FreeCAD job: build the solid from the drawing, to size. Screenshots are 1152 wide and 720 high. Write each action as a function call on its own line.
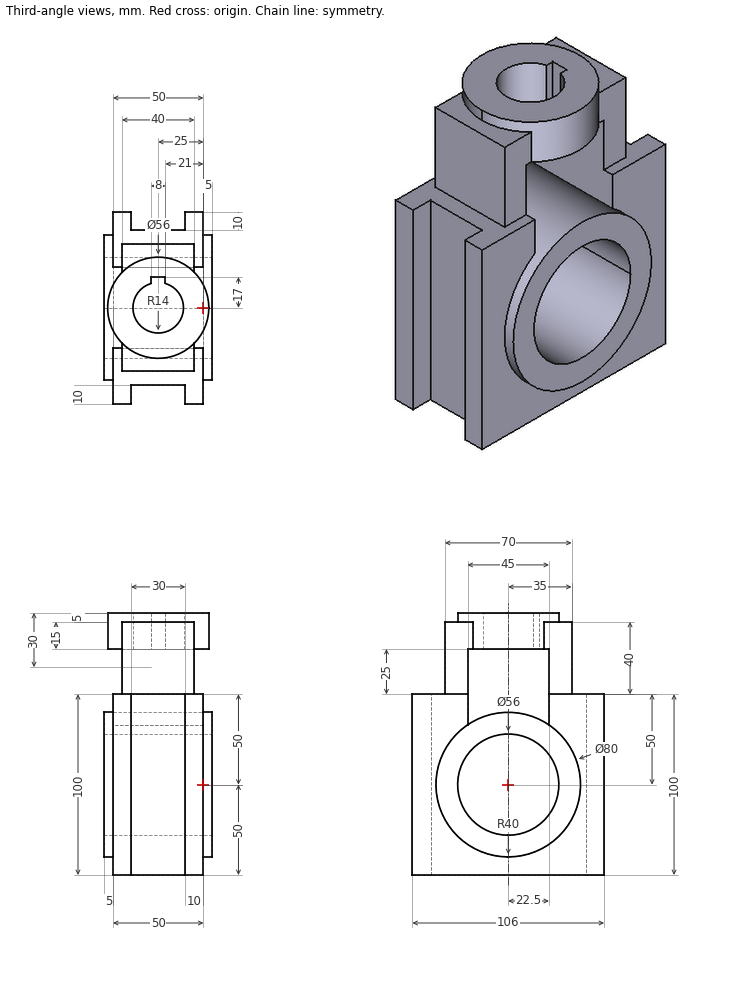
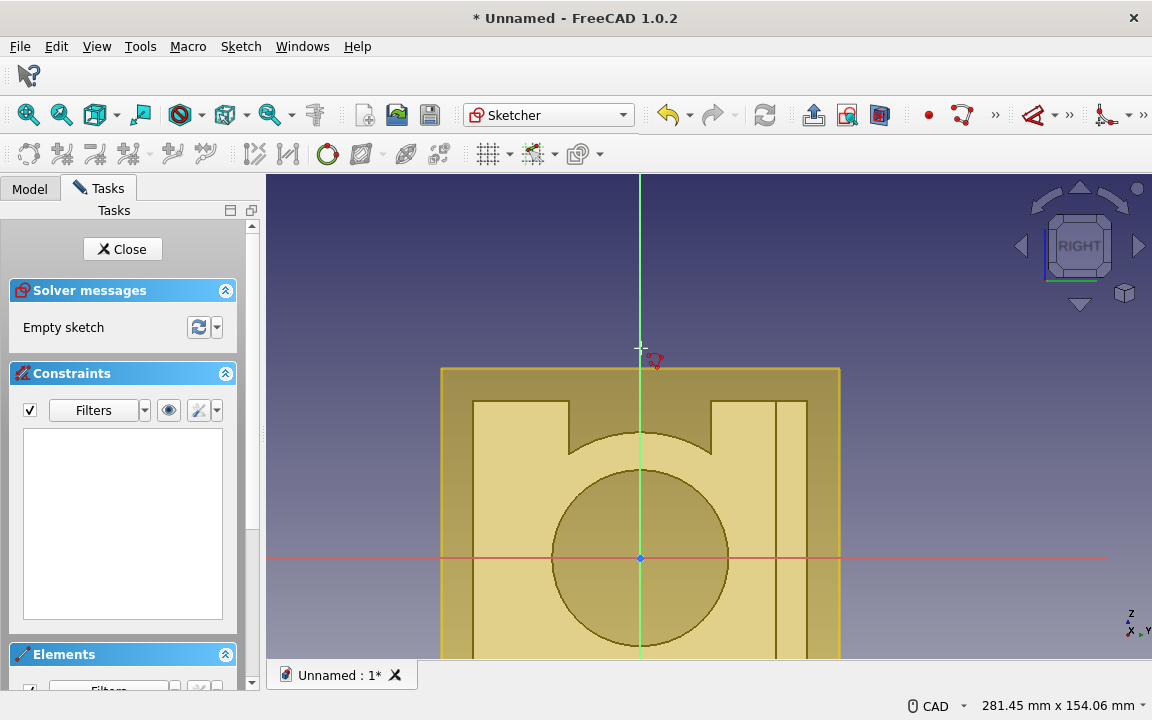
click(569, 401)
click(569, 322)
click(711, 322)
click(711, 401)
click(750, 401)
click(750, 275)
click(530, 275)
click(530, 401)
click(569, 402)
key(Escape)
key(Escape)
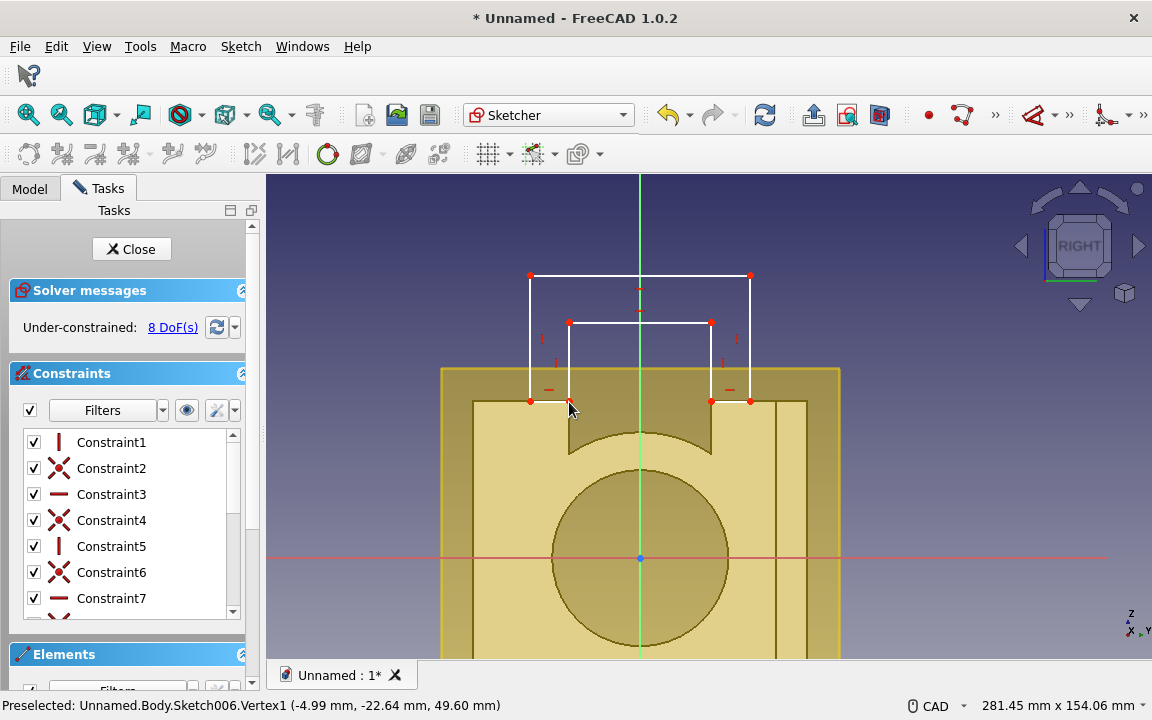
click(569, 402)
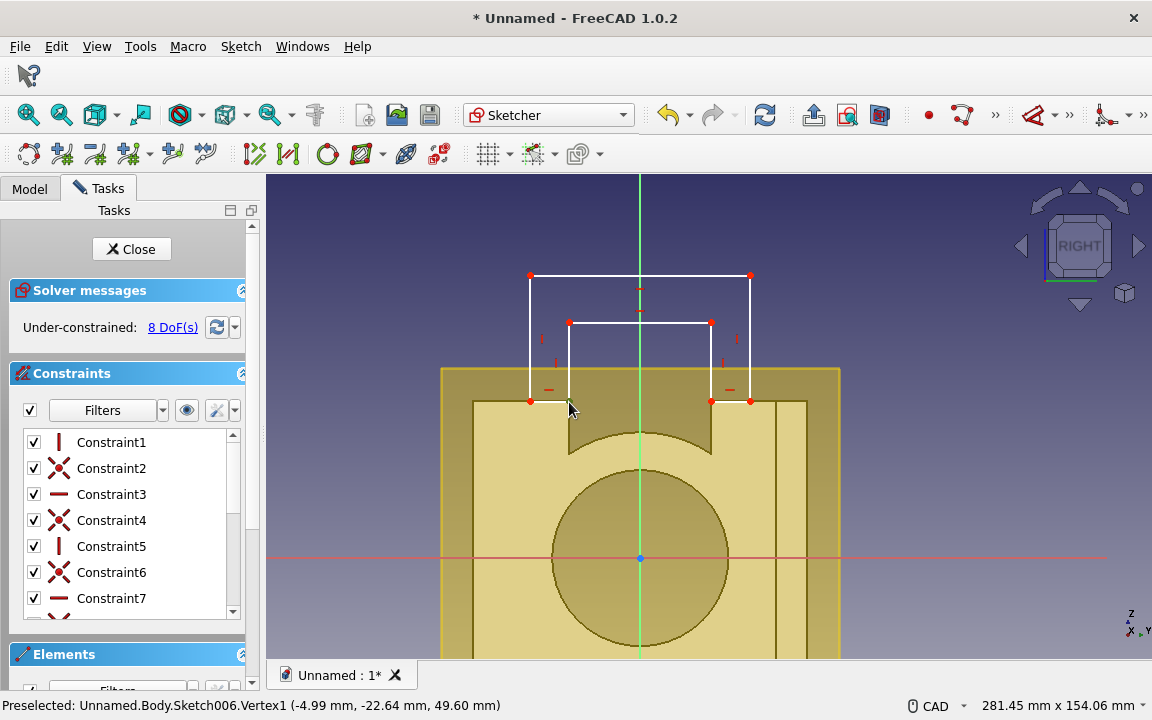
click(711, 402)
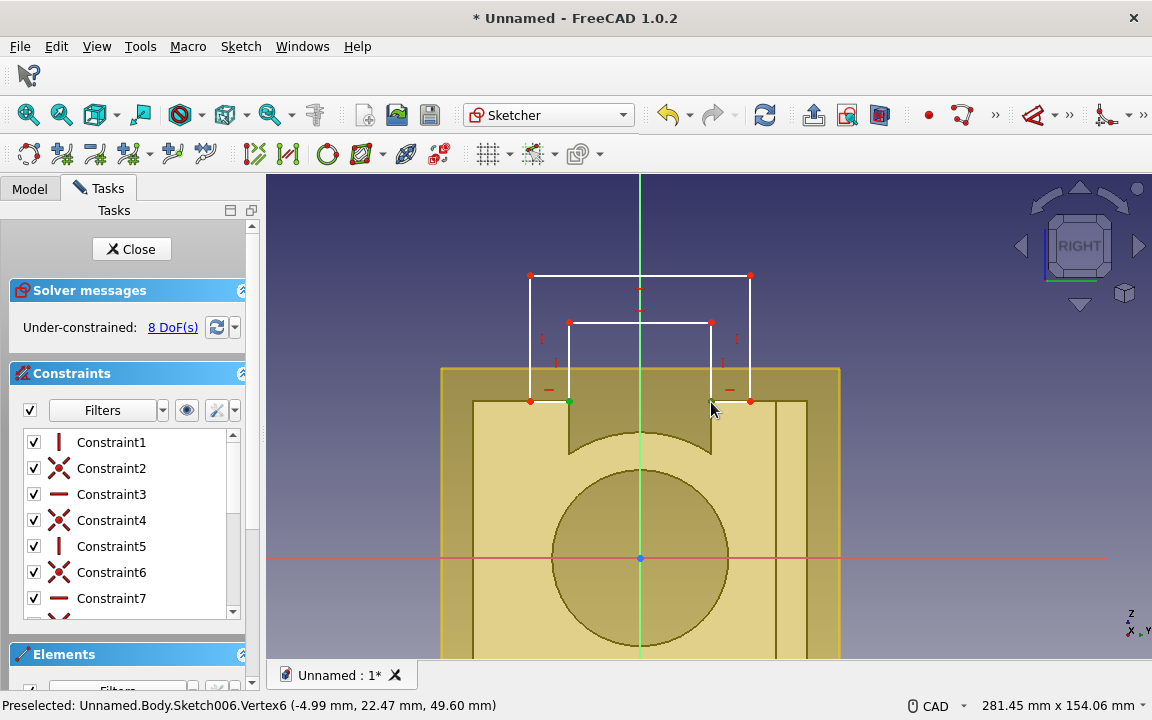
click(640, 600)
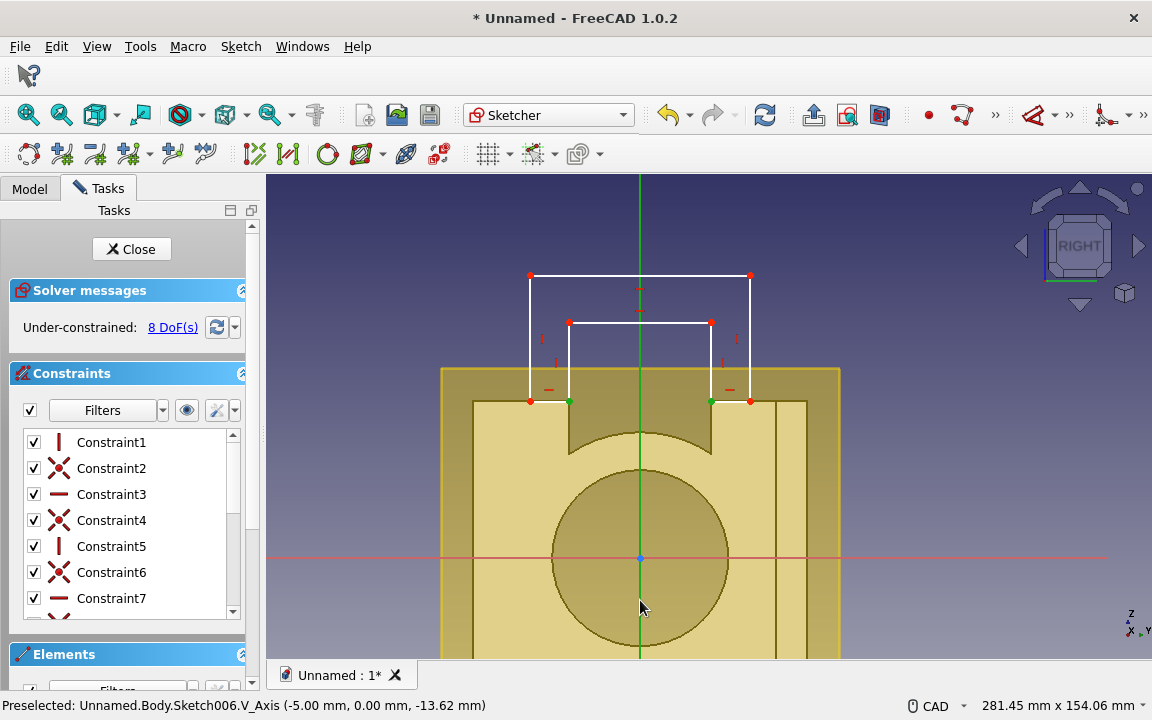
key(s)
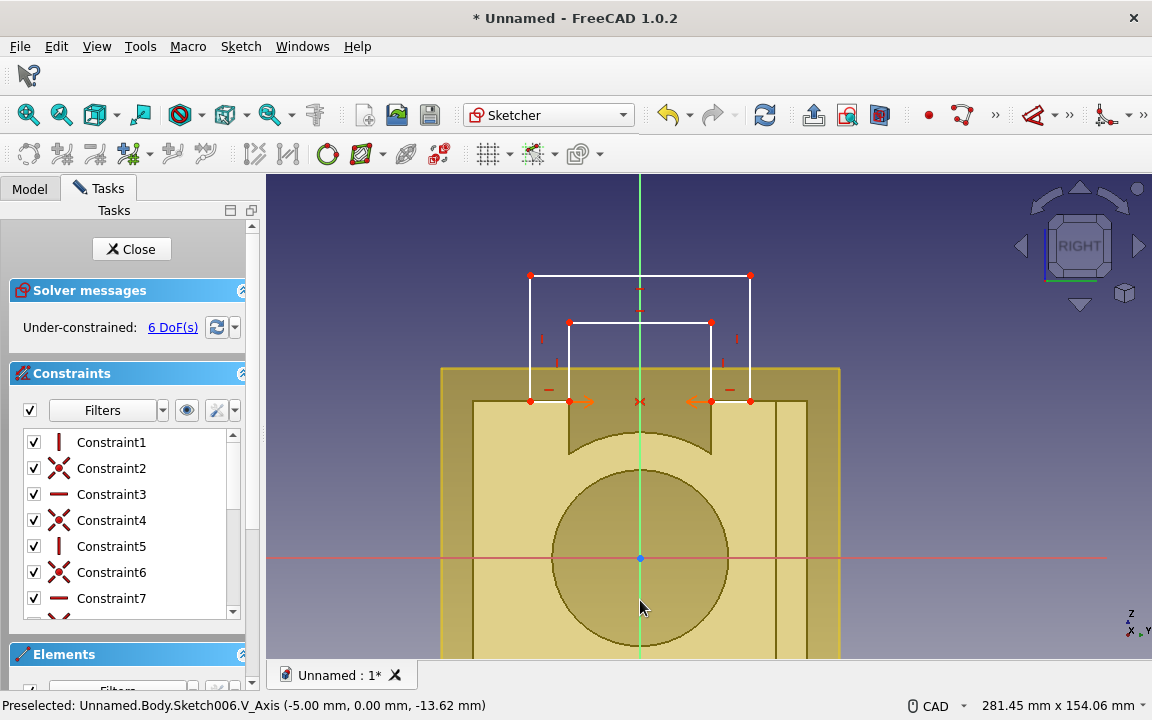
key(d)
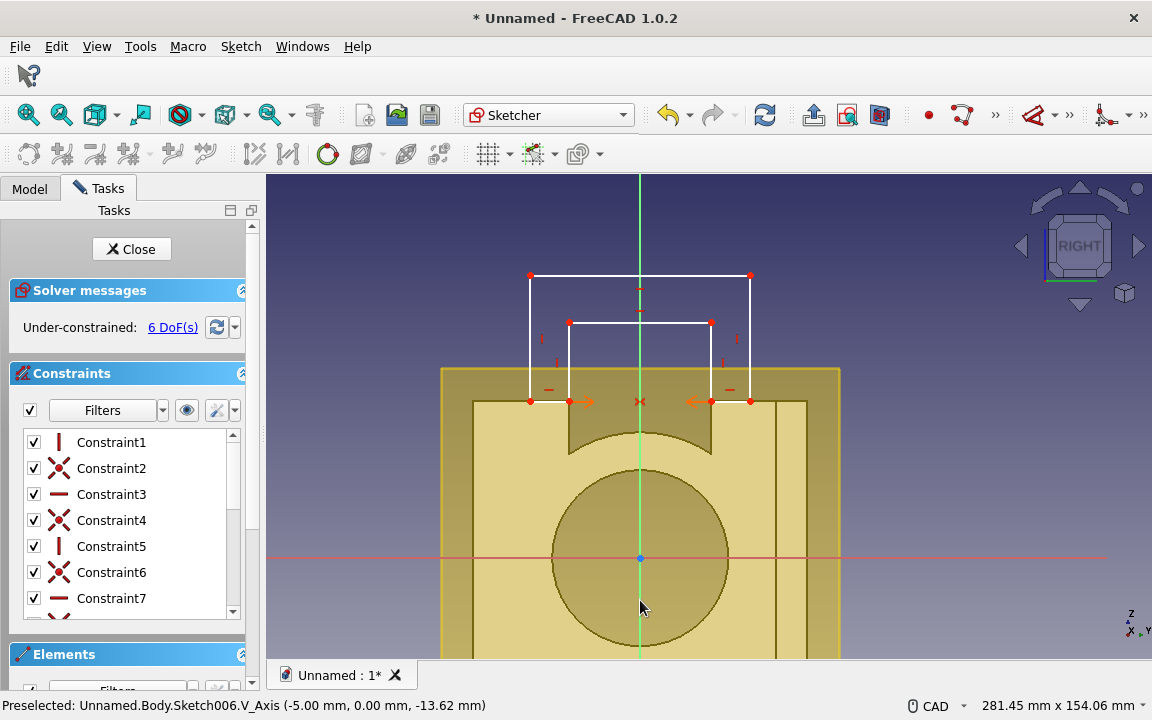
click(569, 378)
click(603, 362)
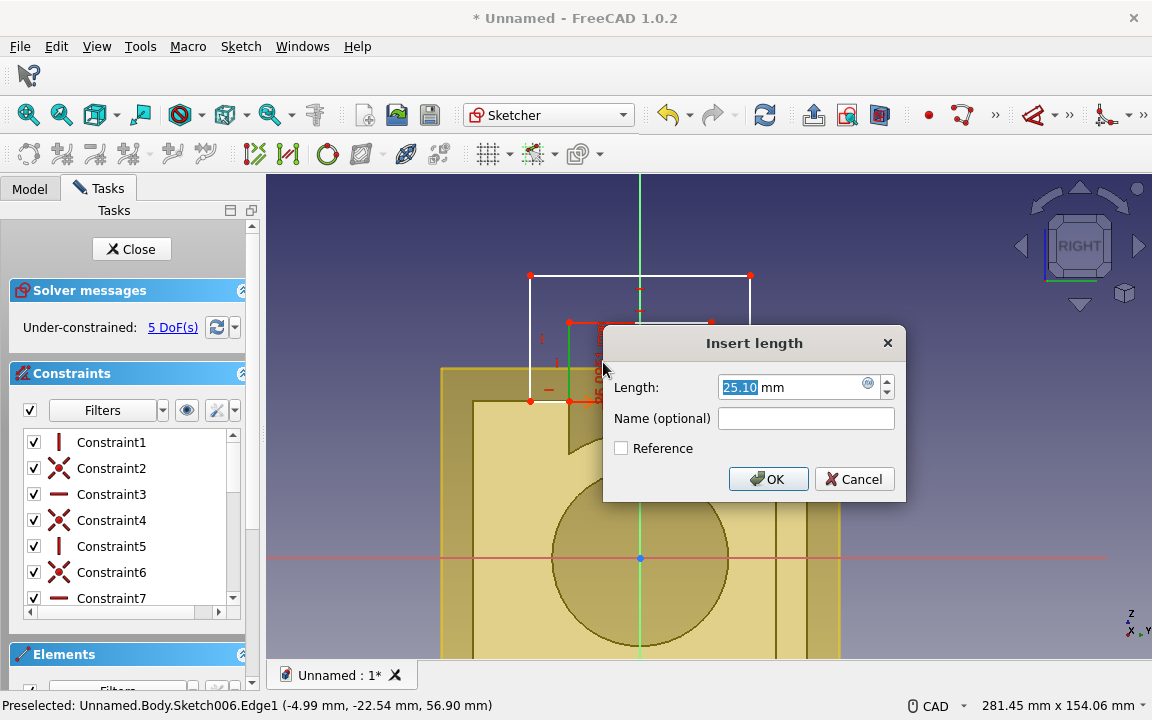
text(25)
key(Return)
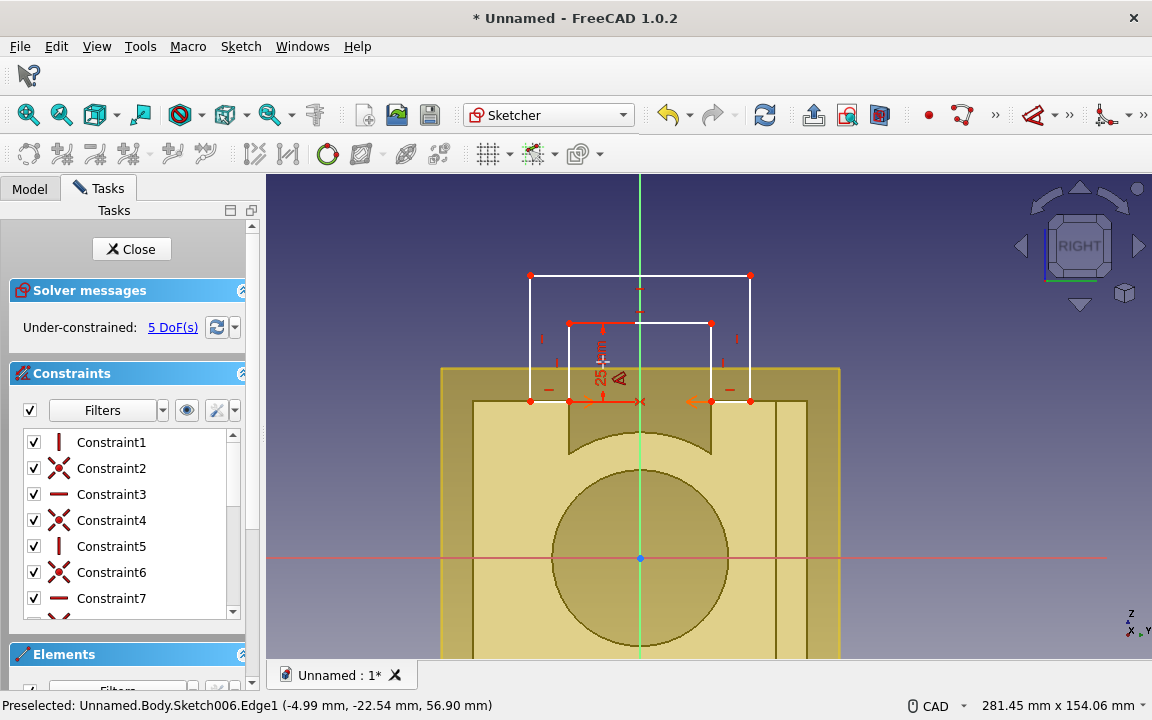
click(612, 323)
click(608, 289)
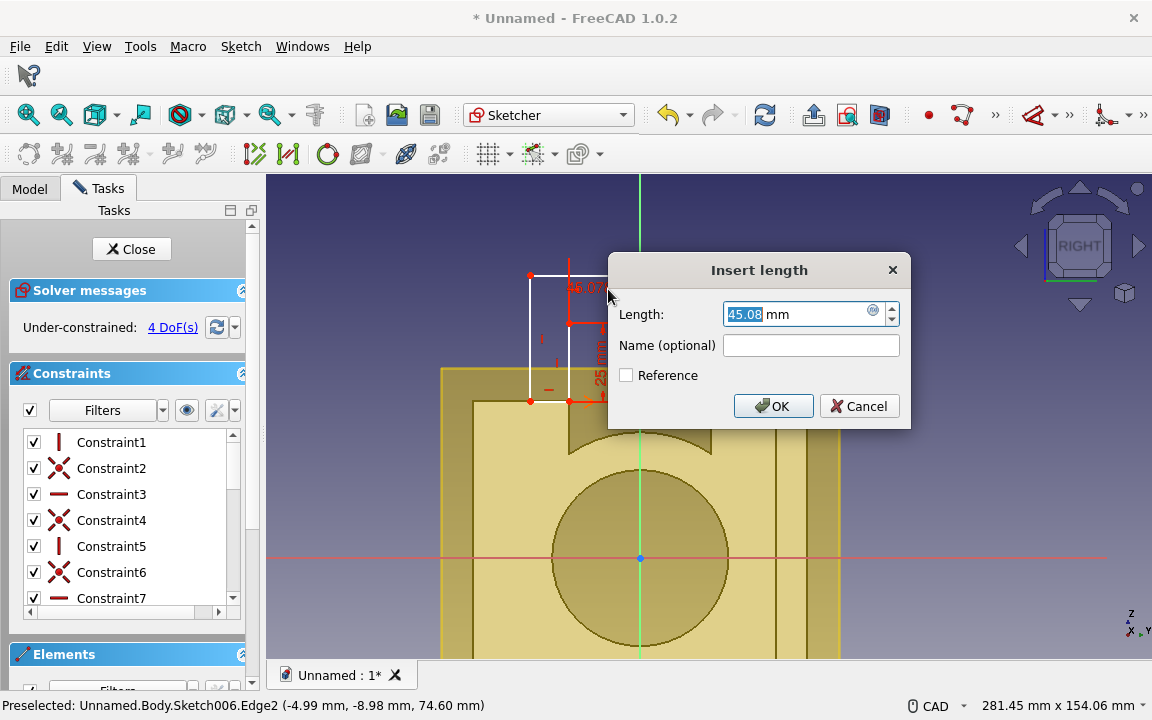
text(45)
key(Return)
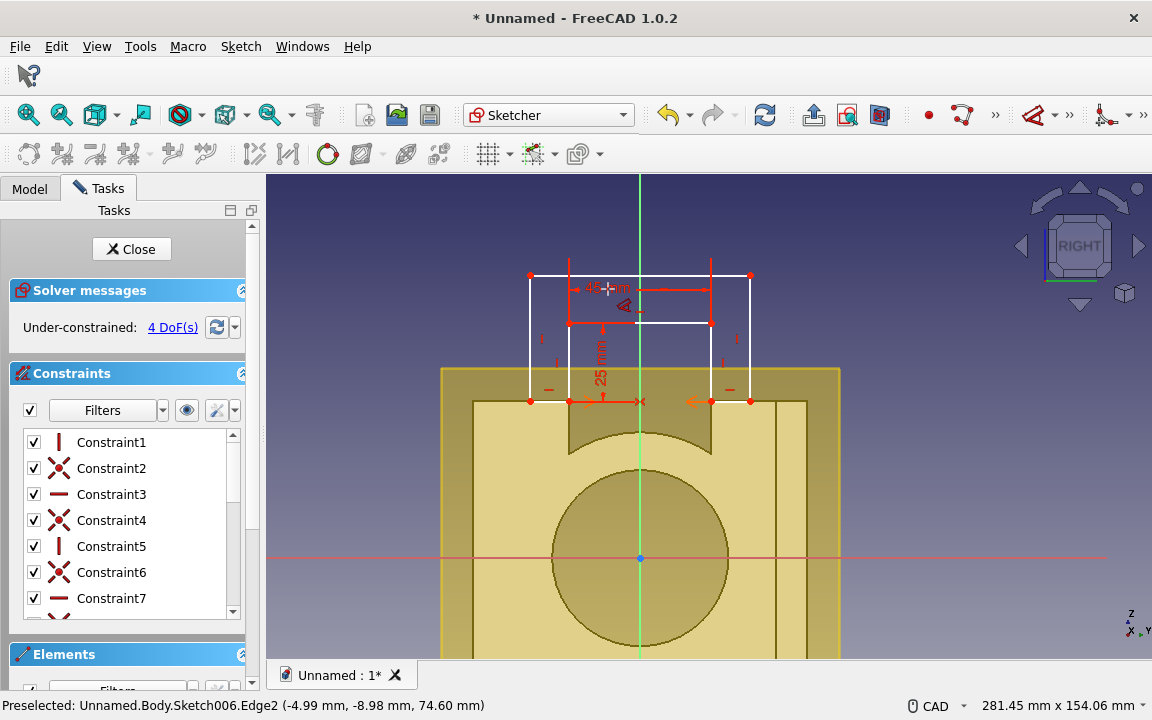
click(750, 364)
click(784, 339)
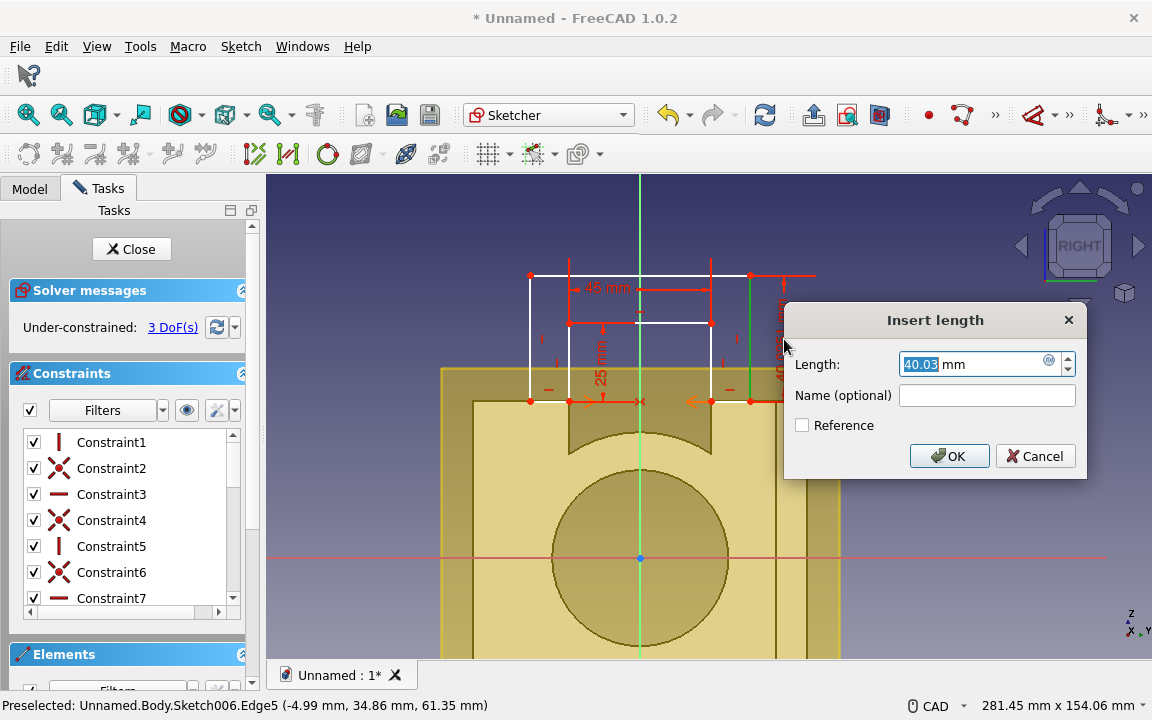
text(40)
key(Return)